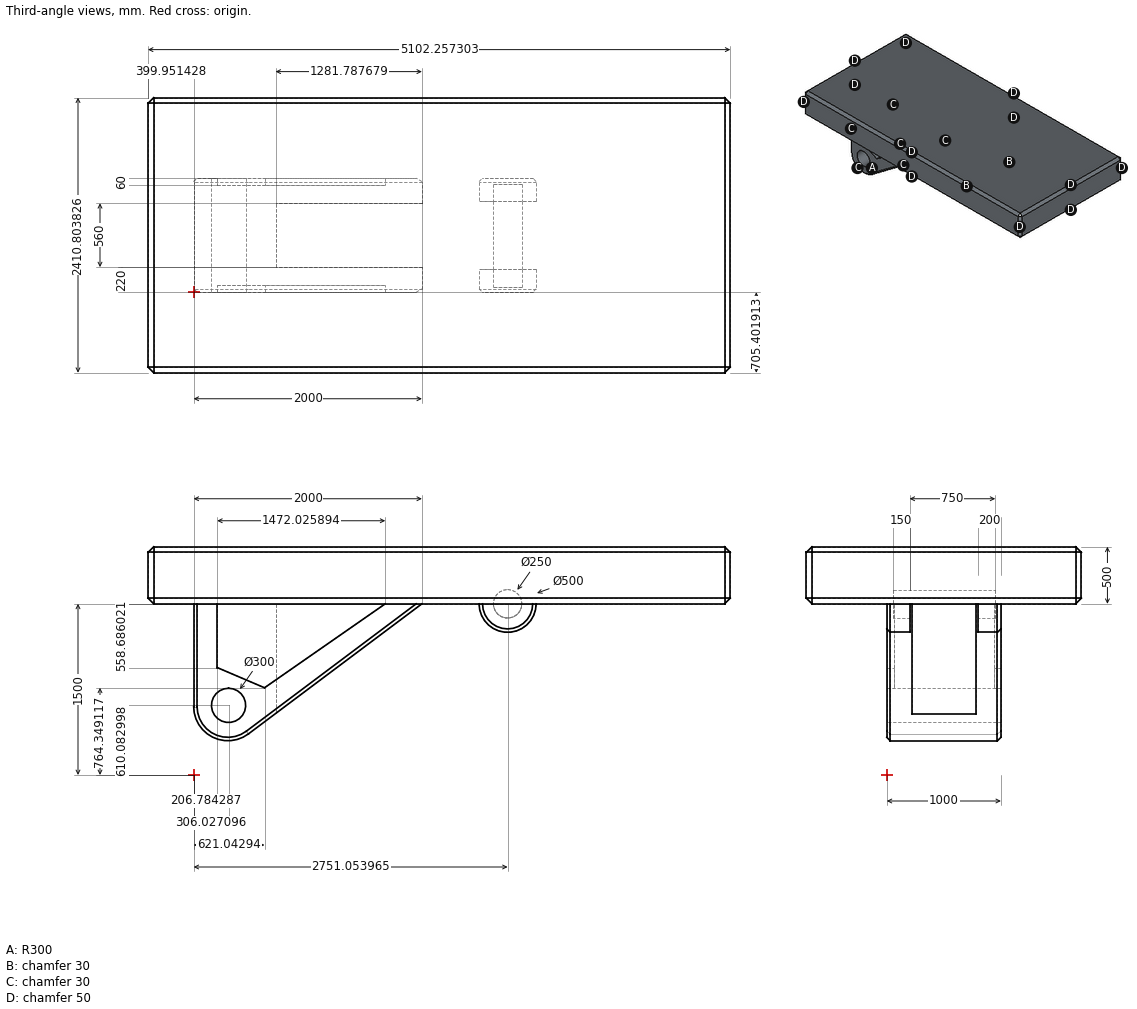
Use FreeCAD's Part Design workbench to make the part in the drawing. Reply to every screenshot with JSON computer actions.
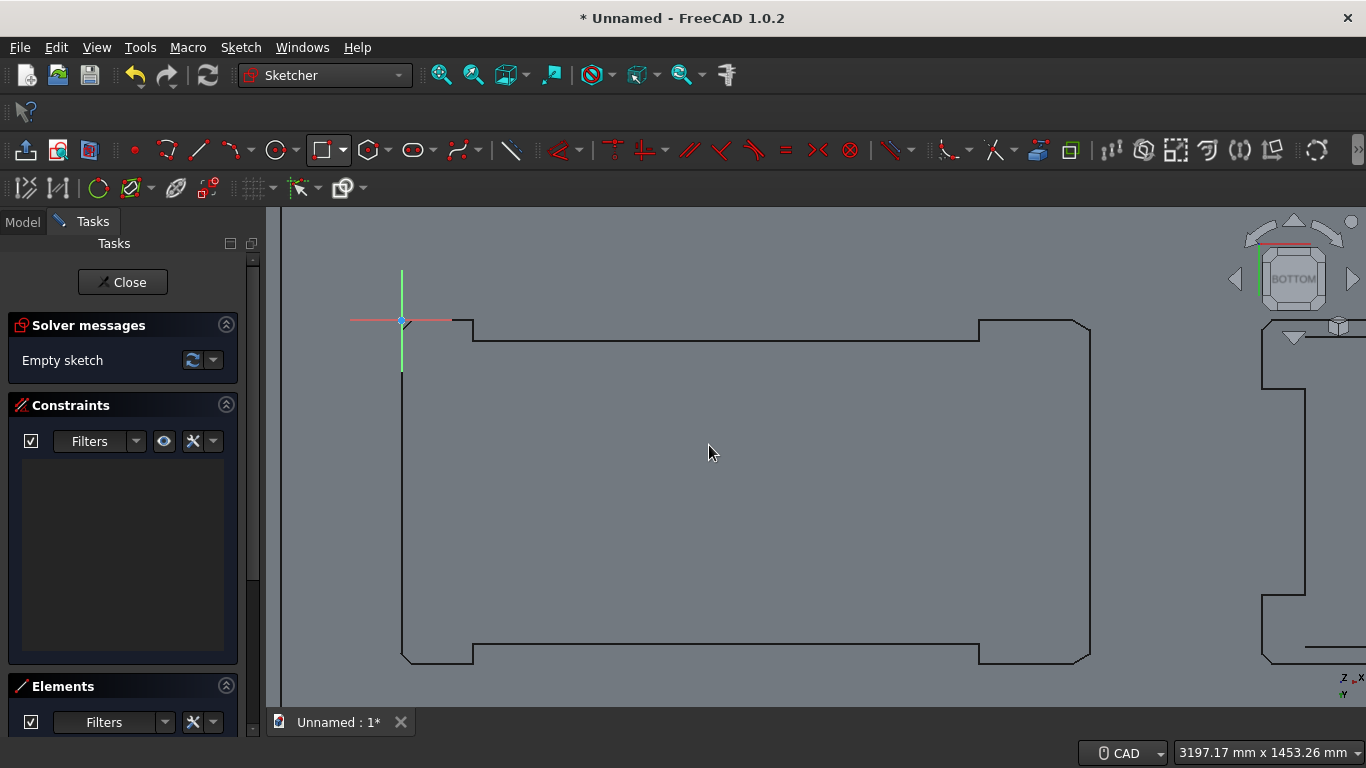
{"action": "left_click", "coordinate": [322, 150]}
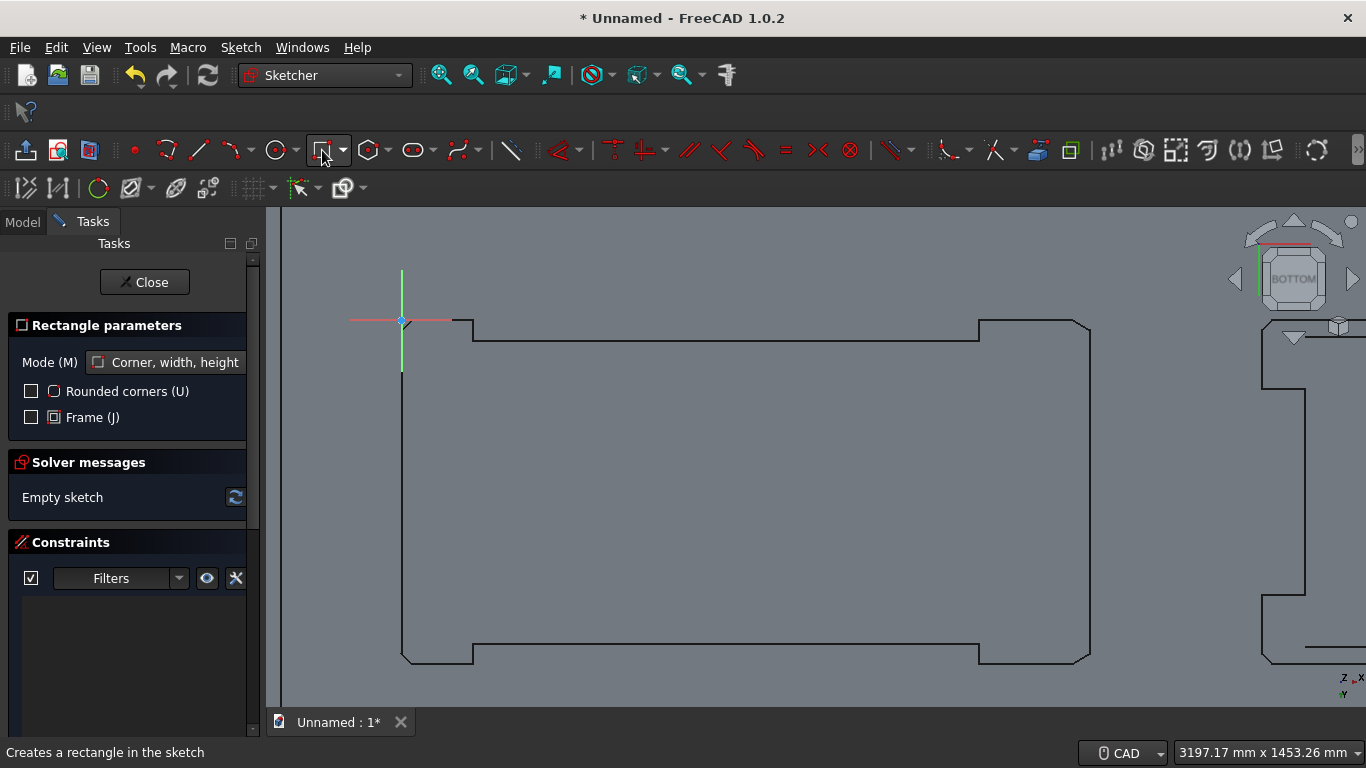
{"action": "left_click", "coordinate": [649, 396]}
{"action": "mouse_move", "coordinate": [1090, 589]}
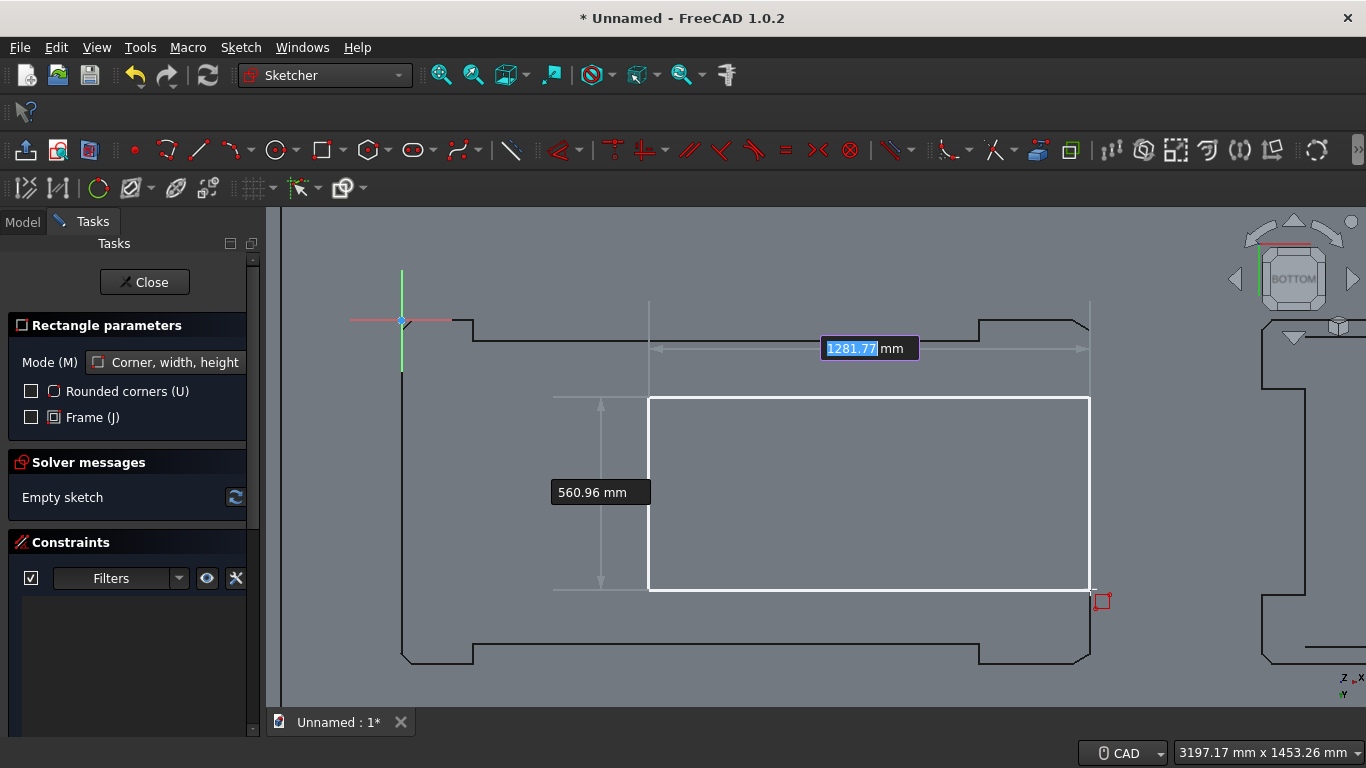
{"action": "type", "text": "1281.787679"}
{"action": "key", "text": "Tab"}
{"action": "type", "text": "560"}
{"action": "key", "text": "Return"}
{"action": "key", "text": "Escape"}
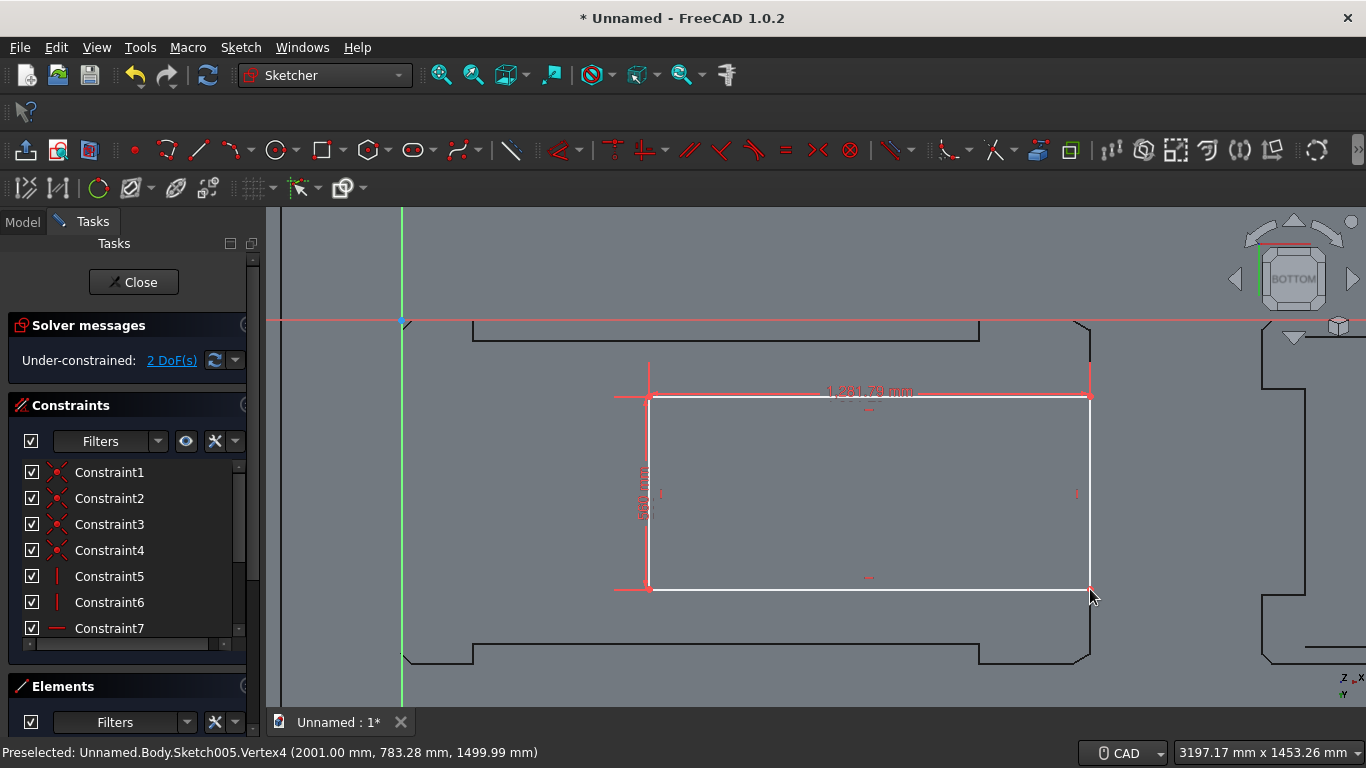
{"action": "left_click", "coordinate": [558, 150]}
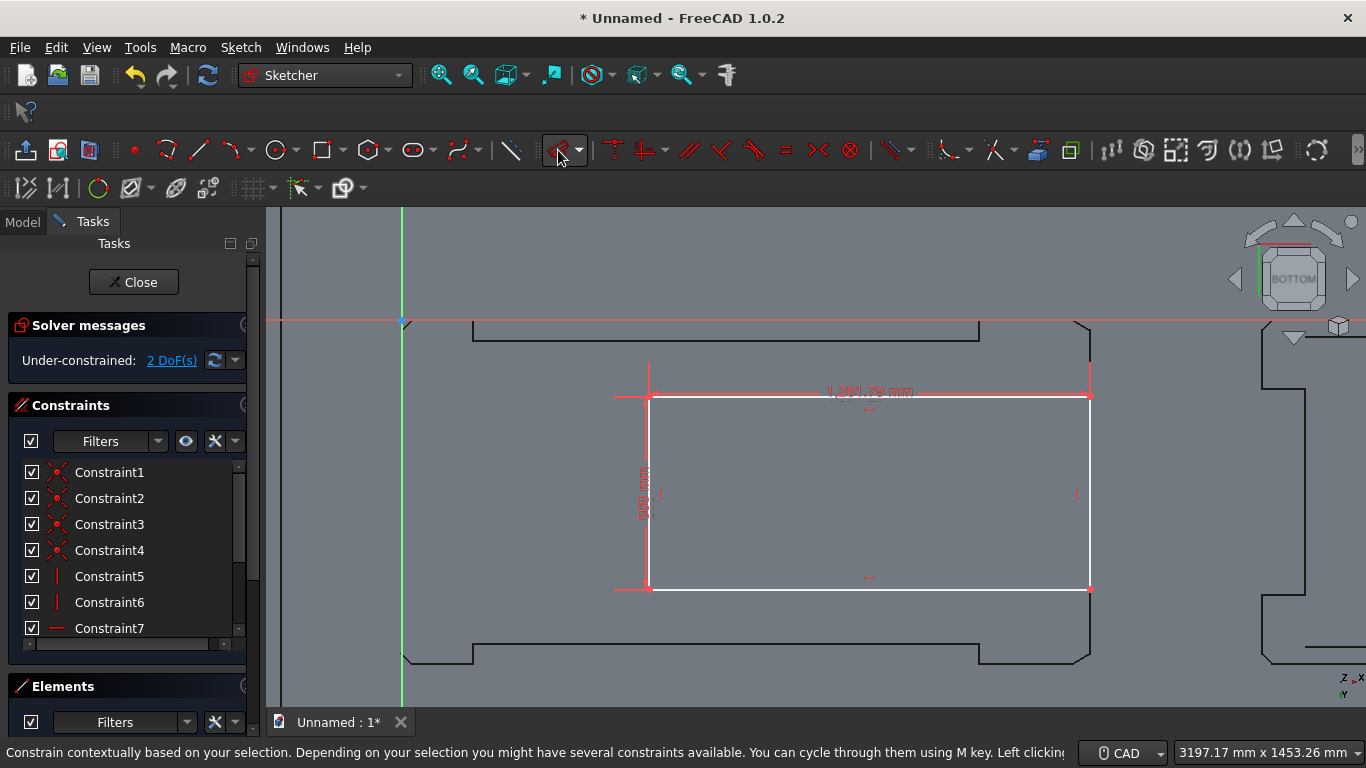
{"action": "left_click", "coordinate": [649, 397]}
{"action": "left_click", "coordinate": [368, 359]}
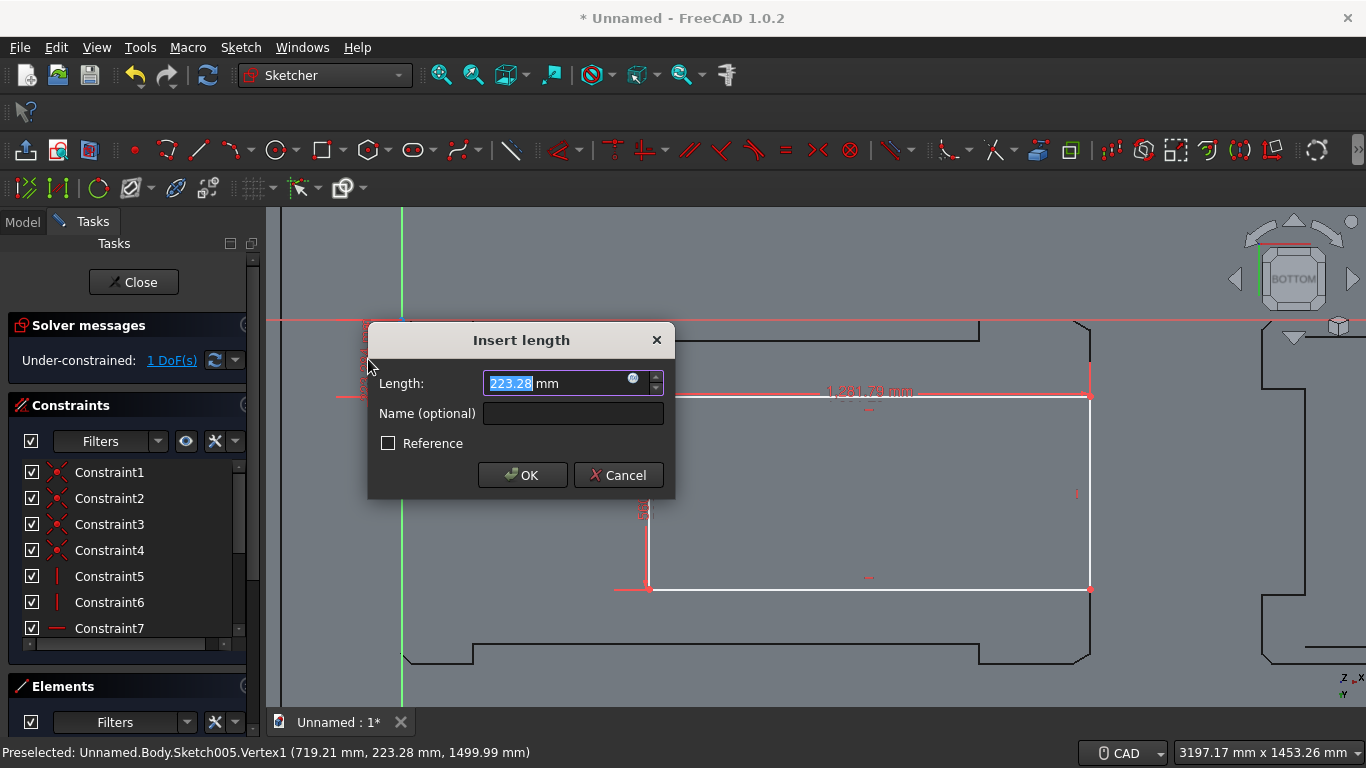
{"action": "type", "text": "220"}
{"action": "key", "text": "Return"}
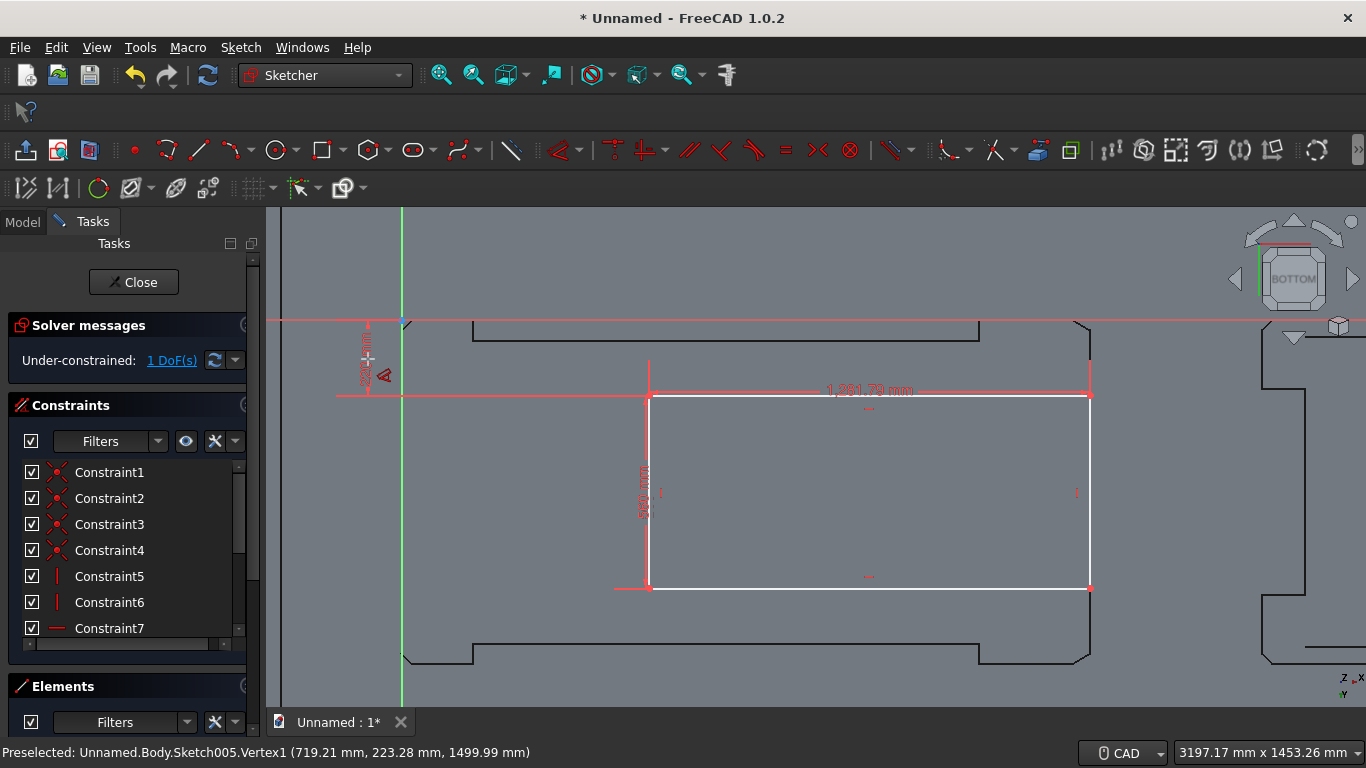
{"action": "left_click", "coordinate": [1090, 589]}
{"action": "left_click", "coordinate": [746, 623]}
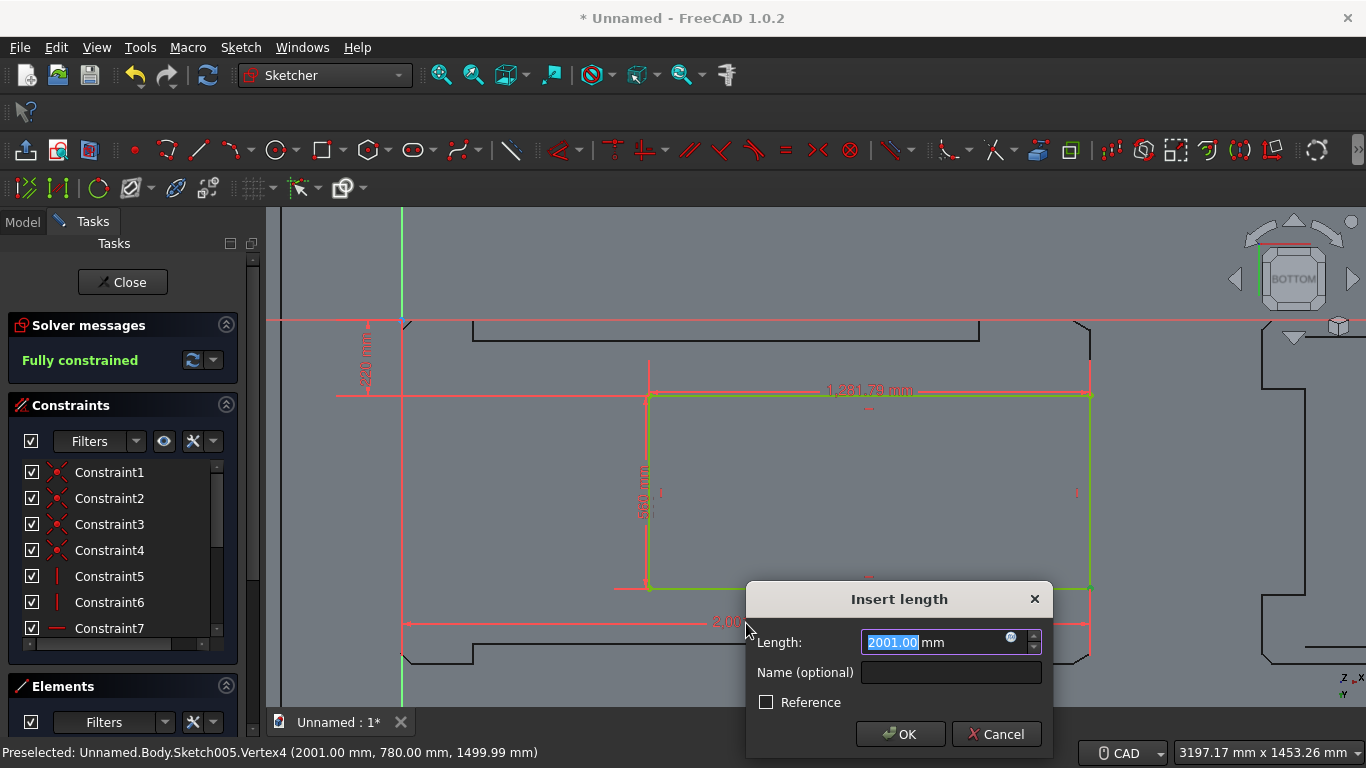
{"action": "type", "text": "2000"}
{"action": "key", "text": "Return"}
{"action": "key", "text": "Escape"}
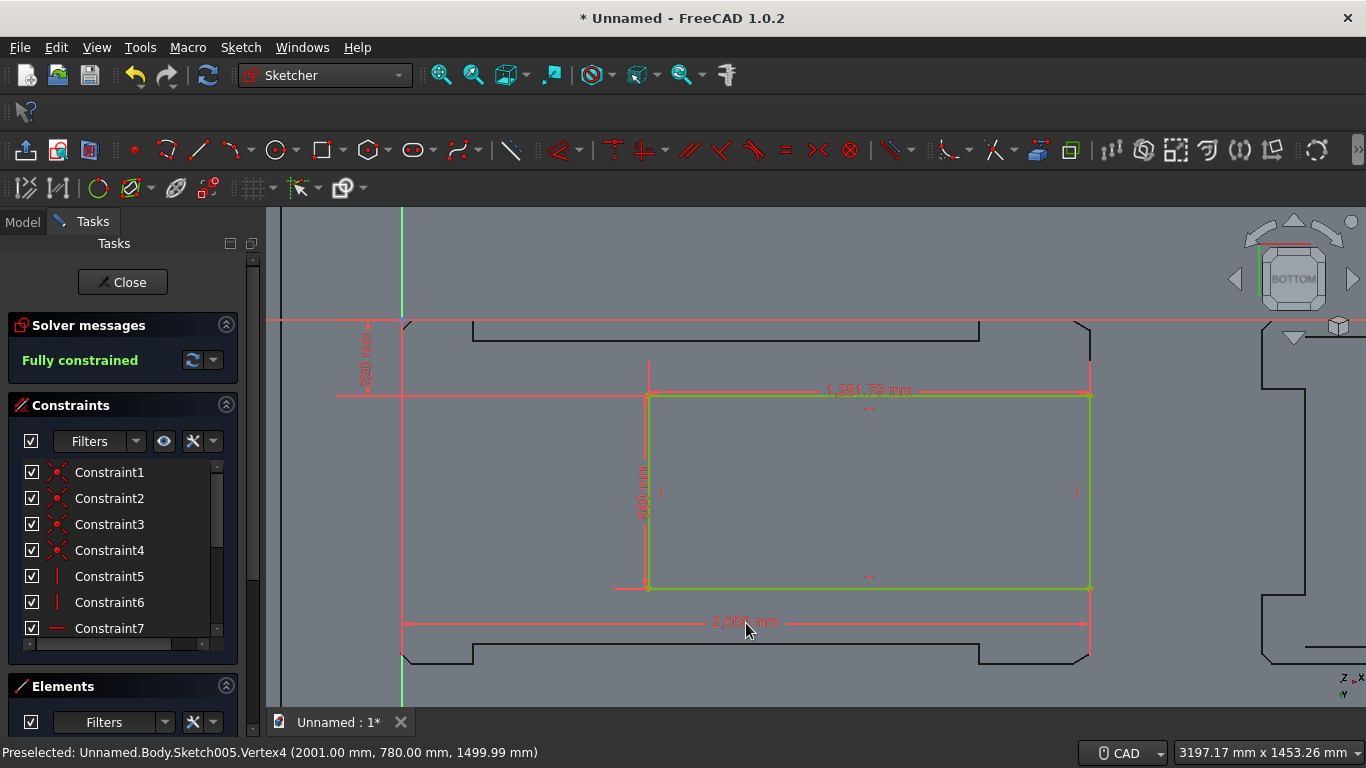
{"action": "left_click", "coordinate": [123, 282]}